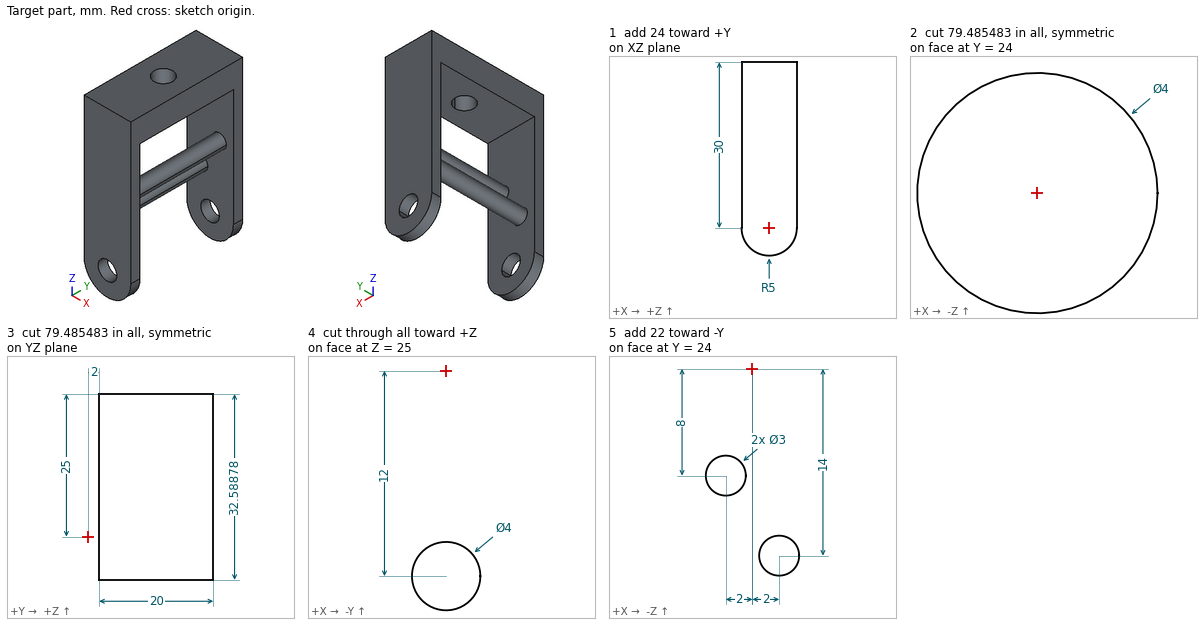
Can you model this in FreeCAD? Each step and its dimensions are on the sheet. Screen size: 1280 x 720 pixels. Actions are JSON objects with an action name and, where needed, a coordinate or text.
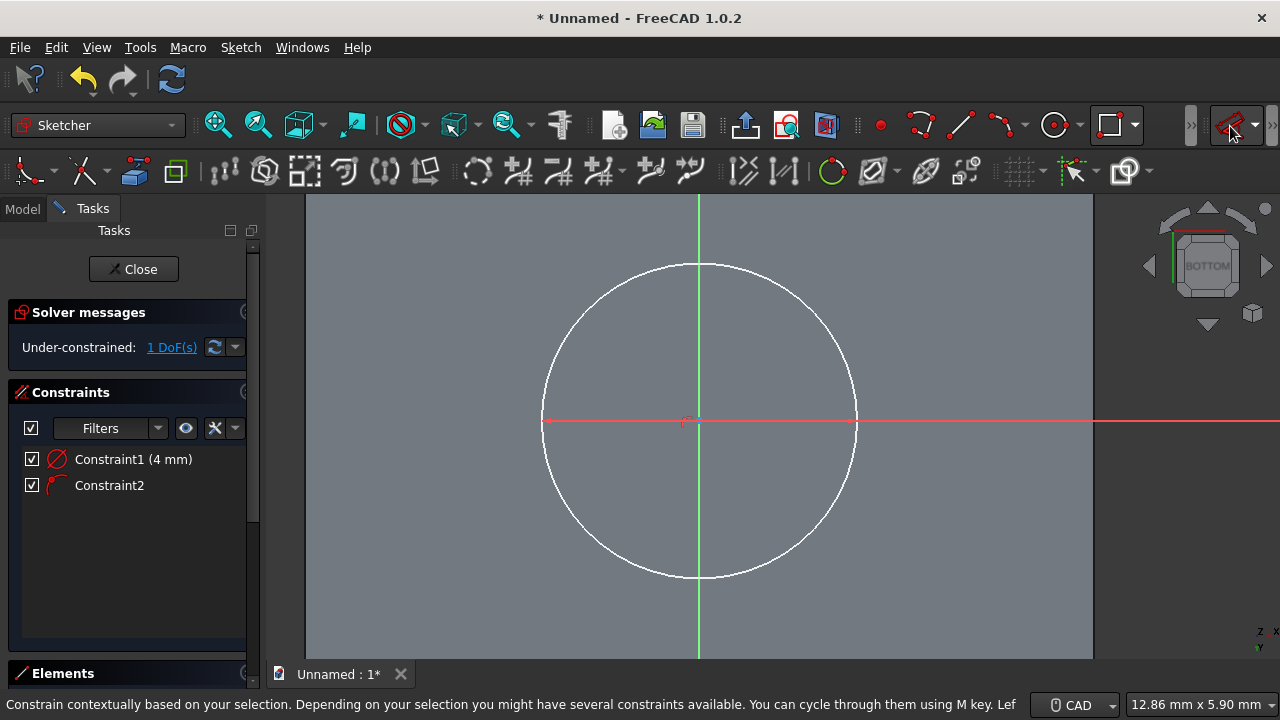
{"action": "left_click", "coordinate": [699, 421]}
{"action": "left_click", "coordinate": [733, 322]}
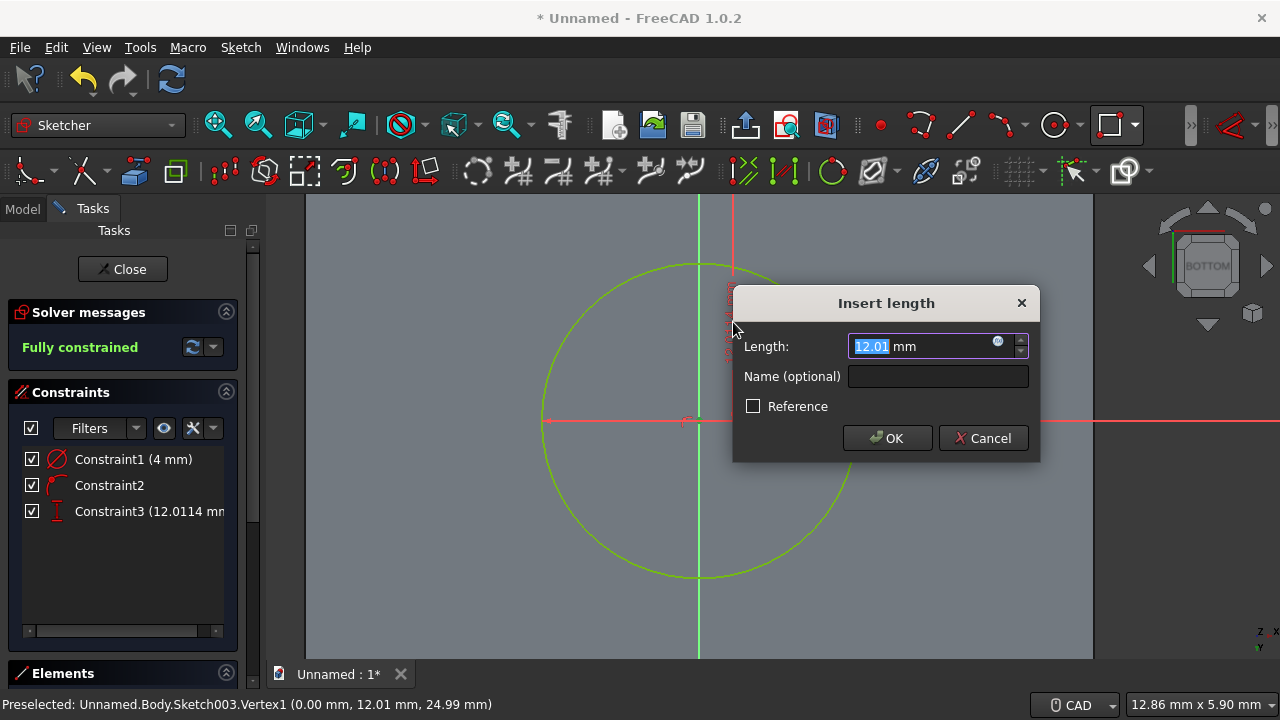
{"action": "type", "text": "12"}
{"action": "key", "text": "Return"}
{"action": "key", "text": "Escape"}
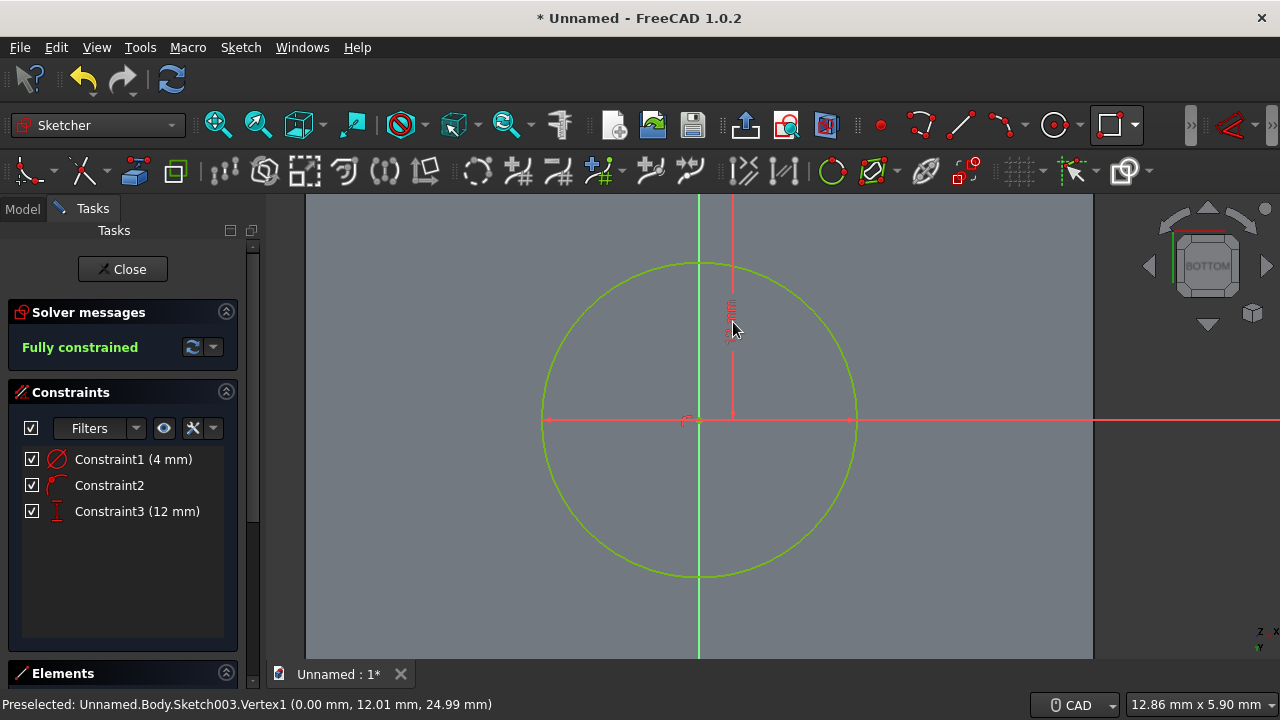
{"action": "left_click", "coordinate": [123, 269]}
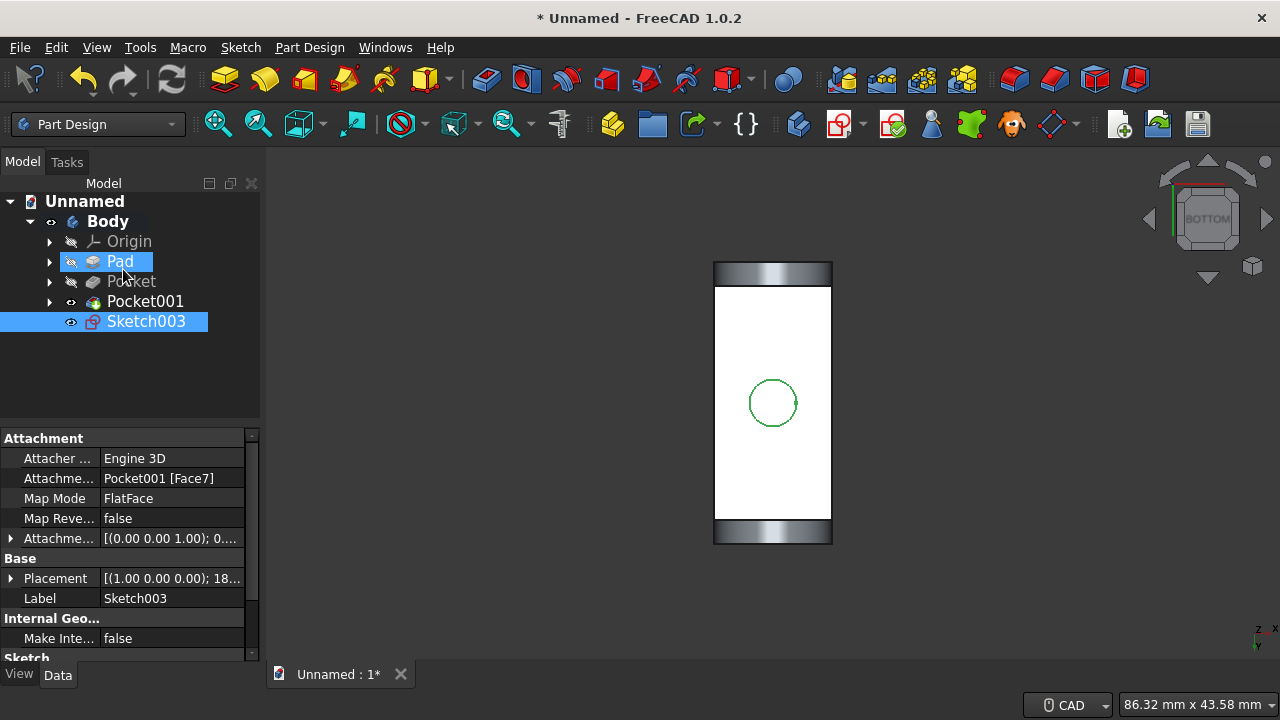
{"action": "left_click", "coordinate": [488, 80]}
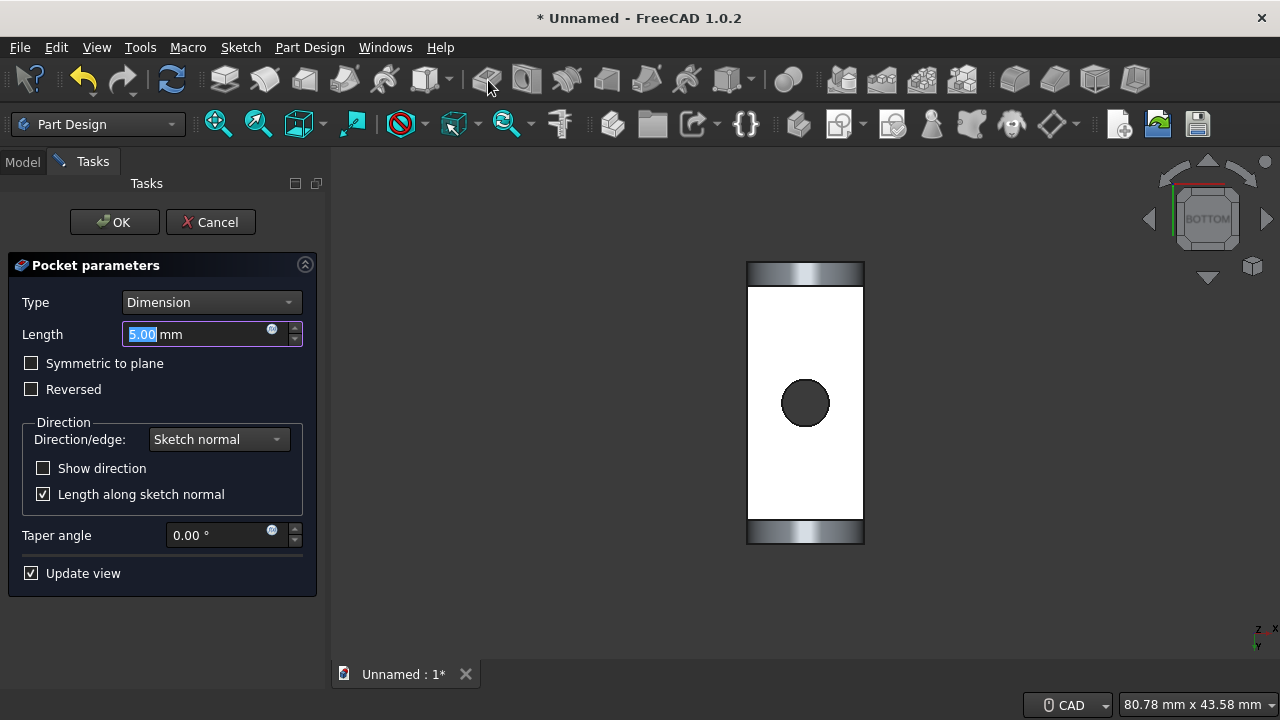
{"action": "left_click", "coordinate": [212, 302]}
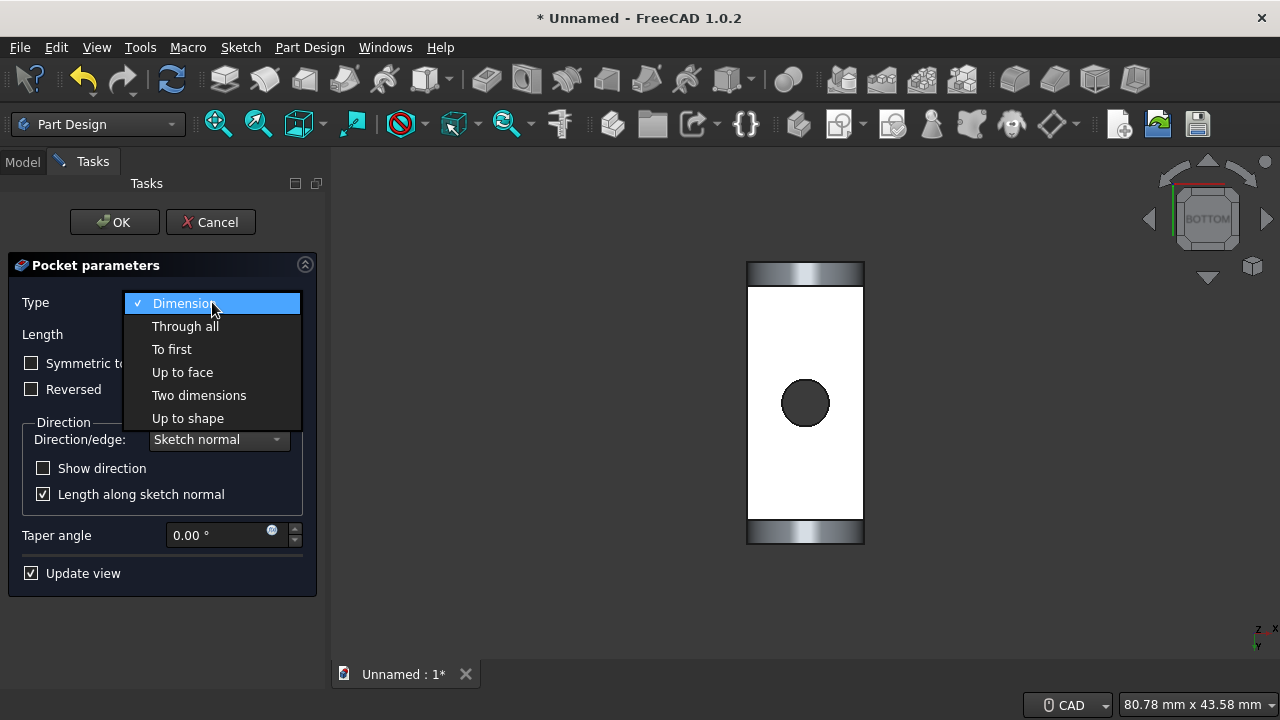
{"action": "left_click", "coordinate": [212, 326]}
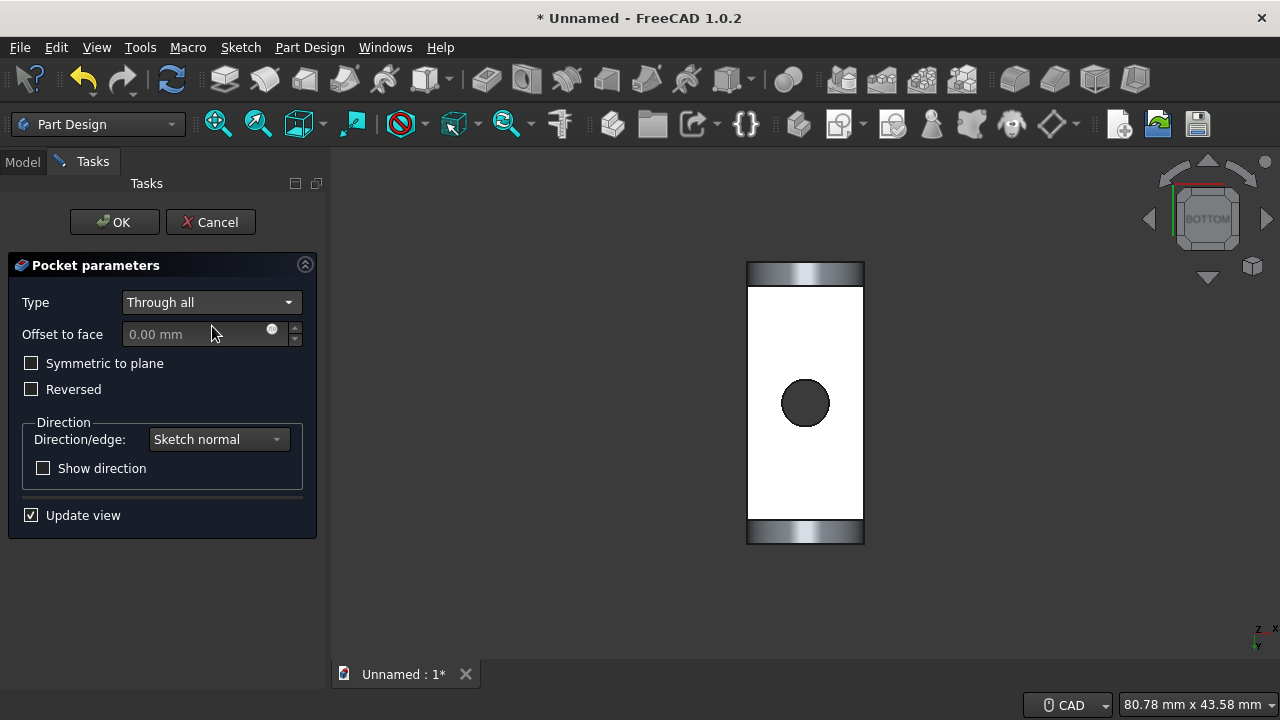
{"action": "left_click", "coordinate": [115, 222]}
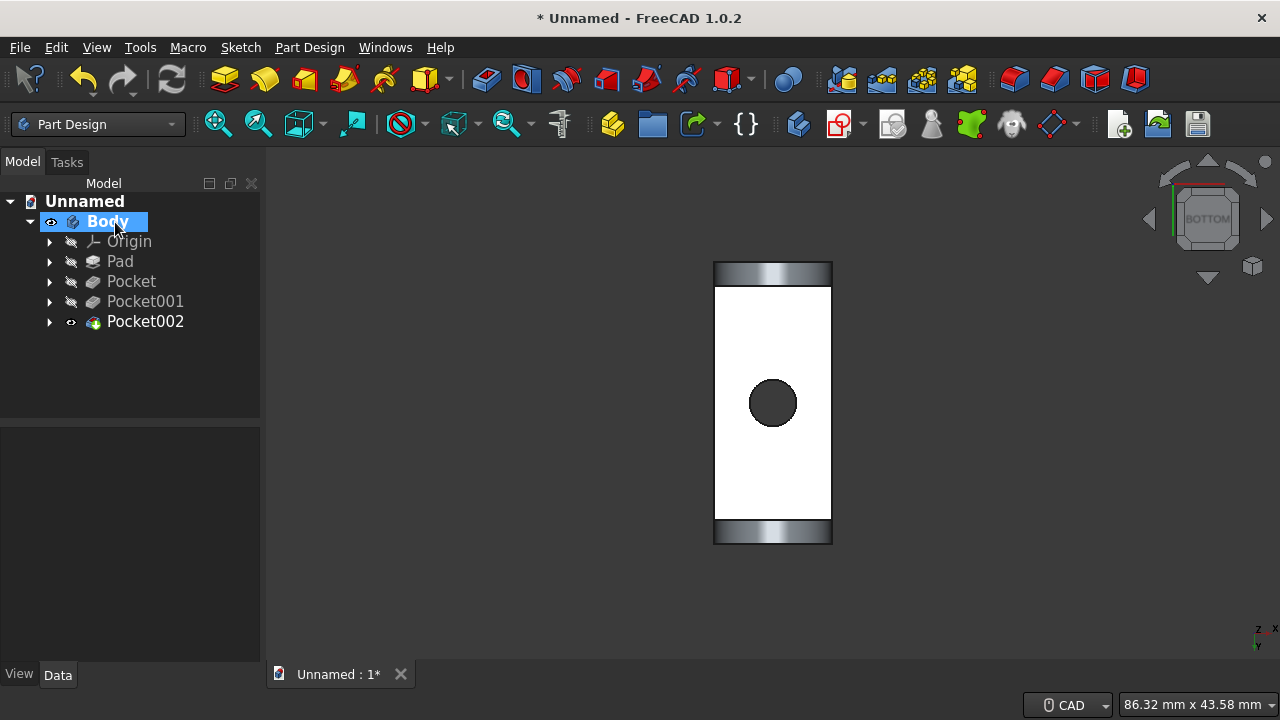
{"action": "key", "text": "4"}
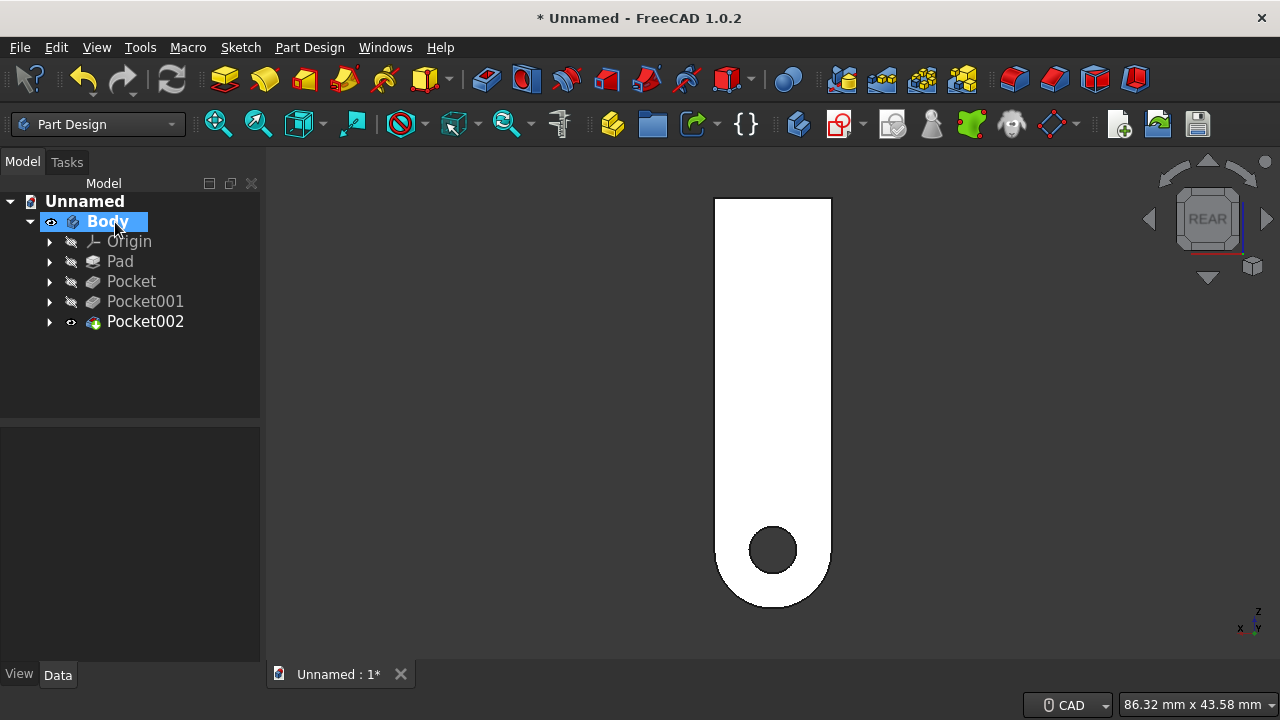
{"action": "left_click", "coordinate": [773, 285]}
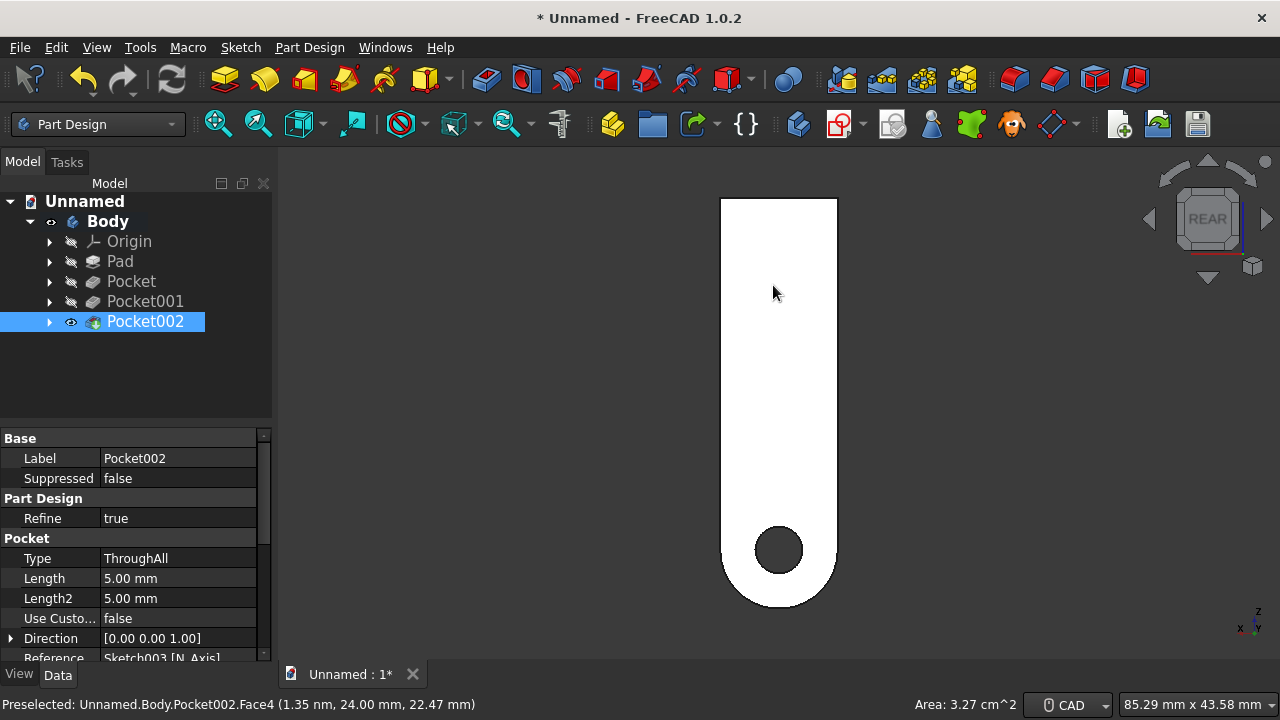
{"action": "left_click", "coordinate": [840, 124]}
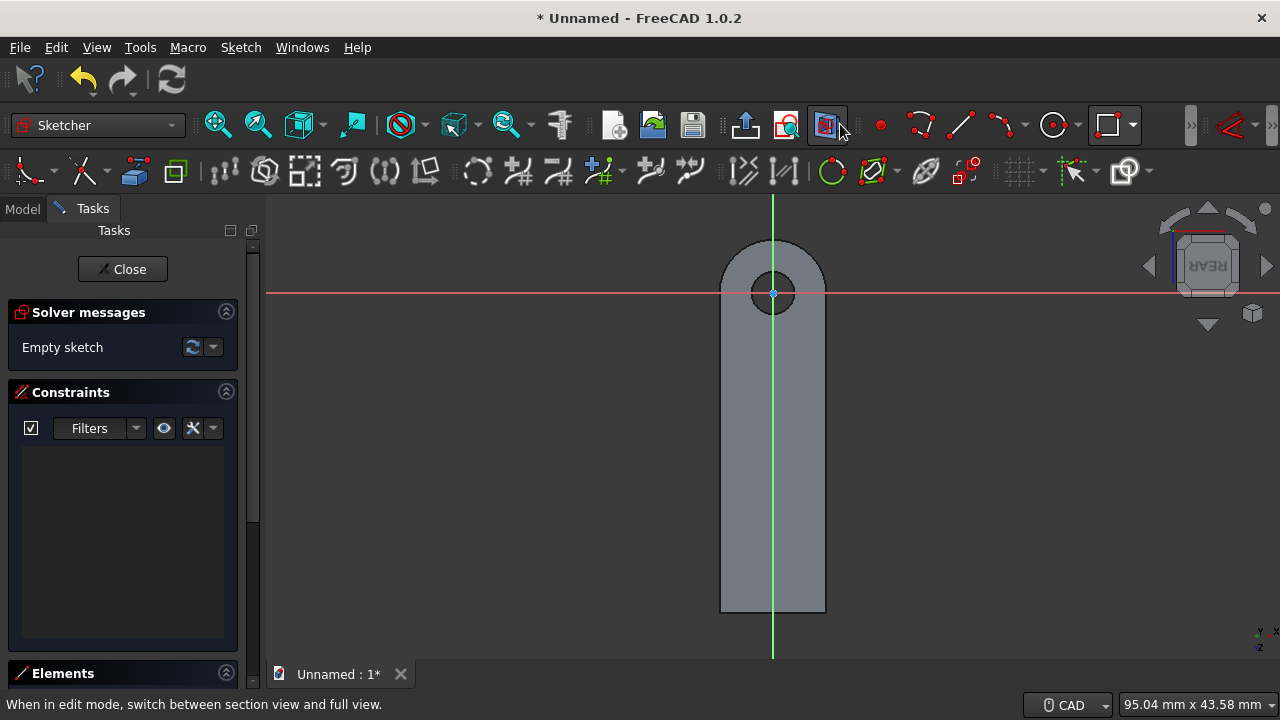
{"action": "scroll", "coordinate": [856, 314], "scroll_direction": "up", "scroll_amount": 3}